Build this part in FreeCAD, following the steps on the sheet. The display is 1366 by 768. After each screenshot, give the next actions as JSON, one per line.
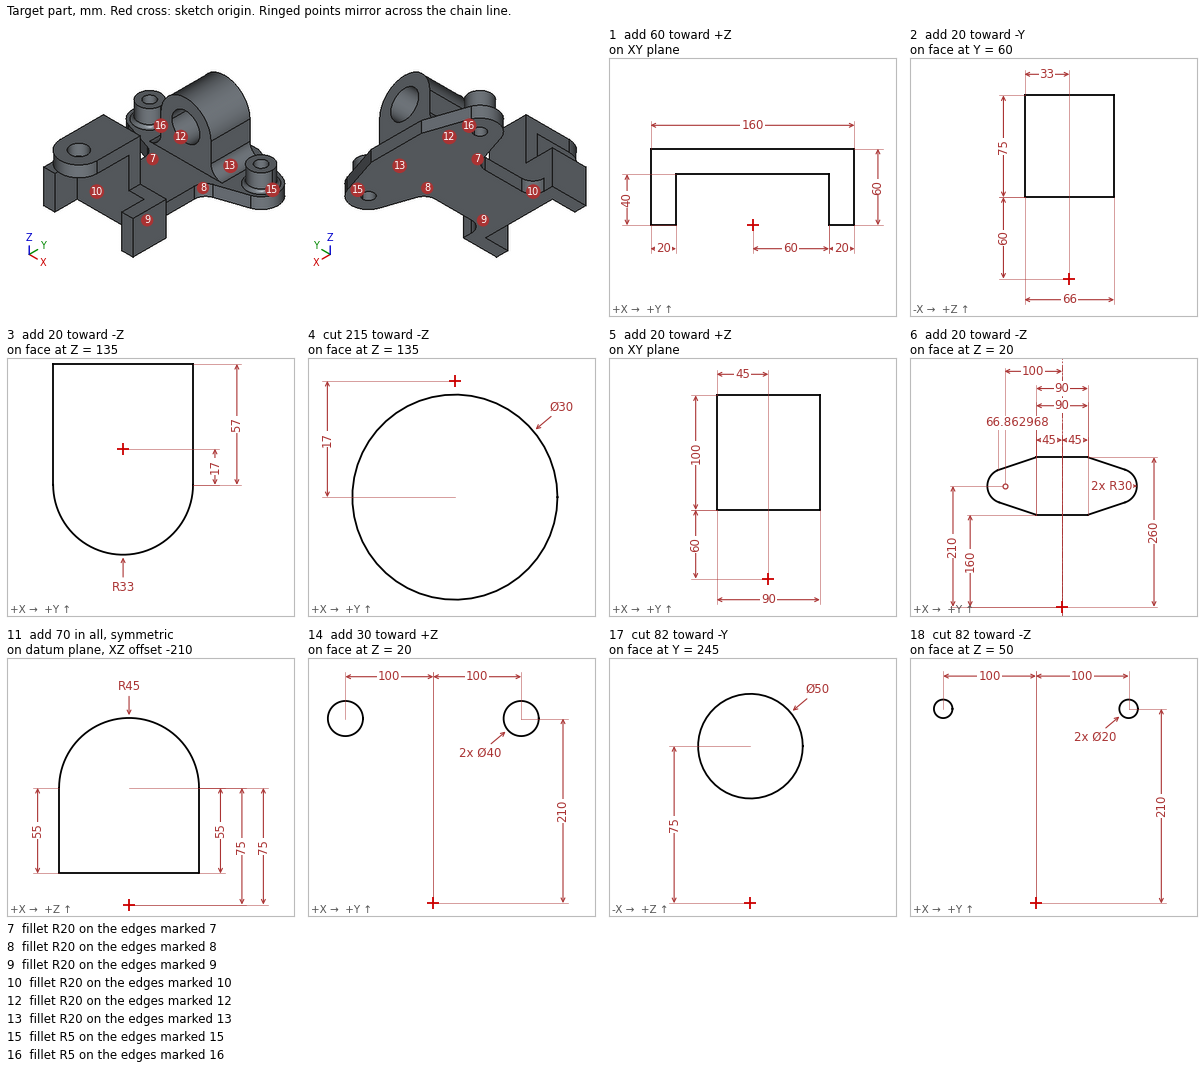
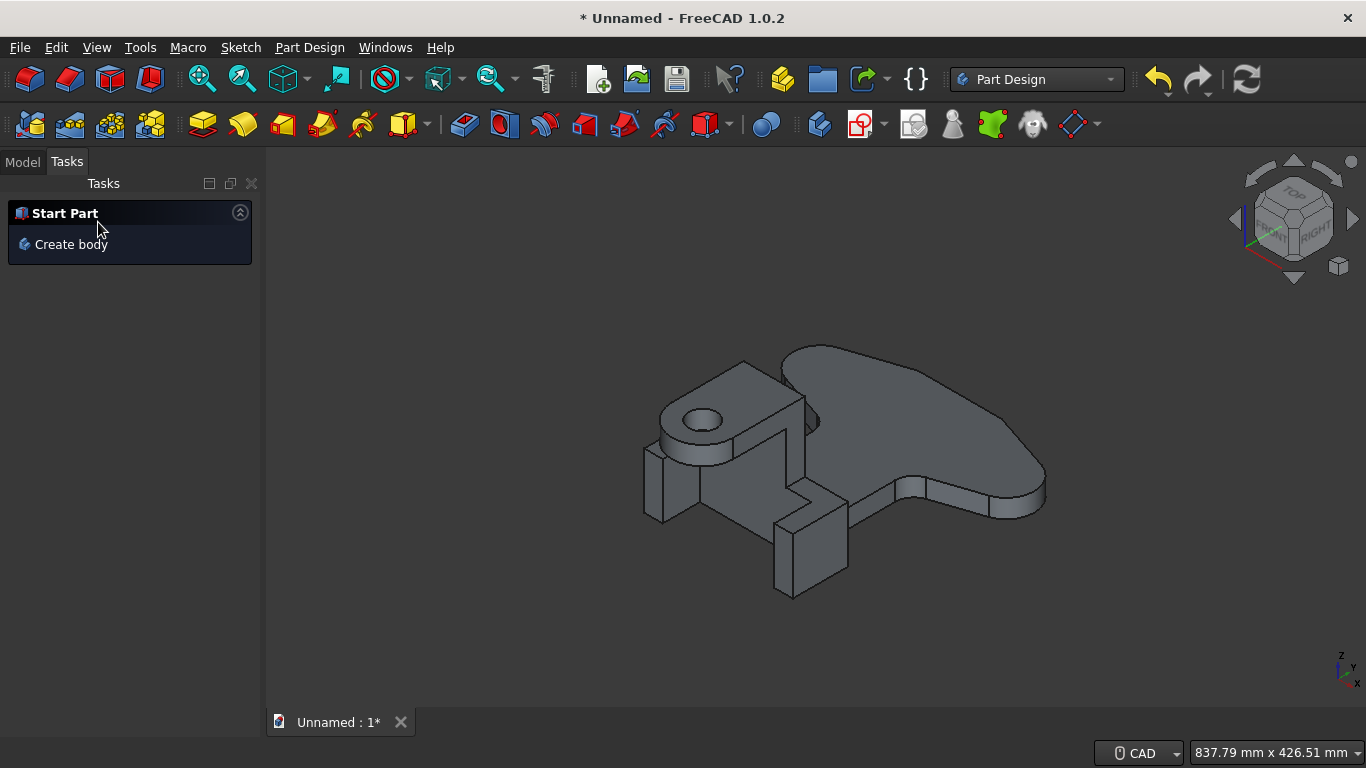
{"action": "key", "text": "2"}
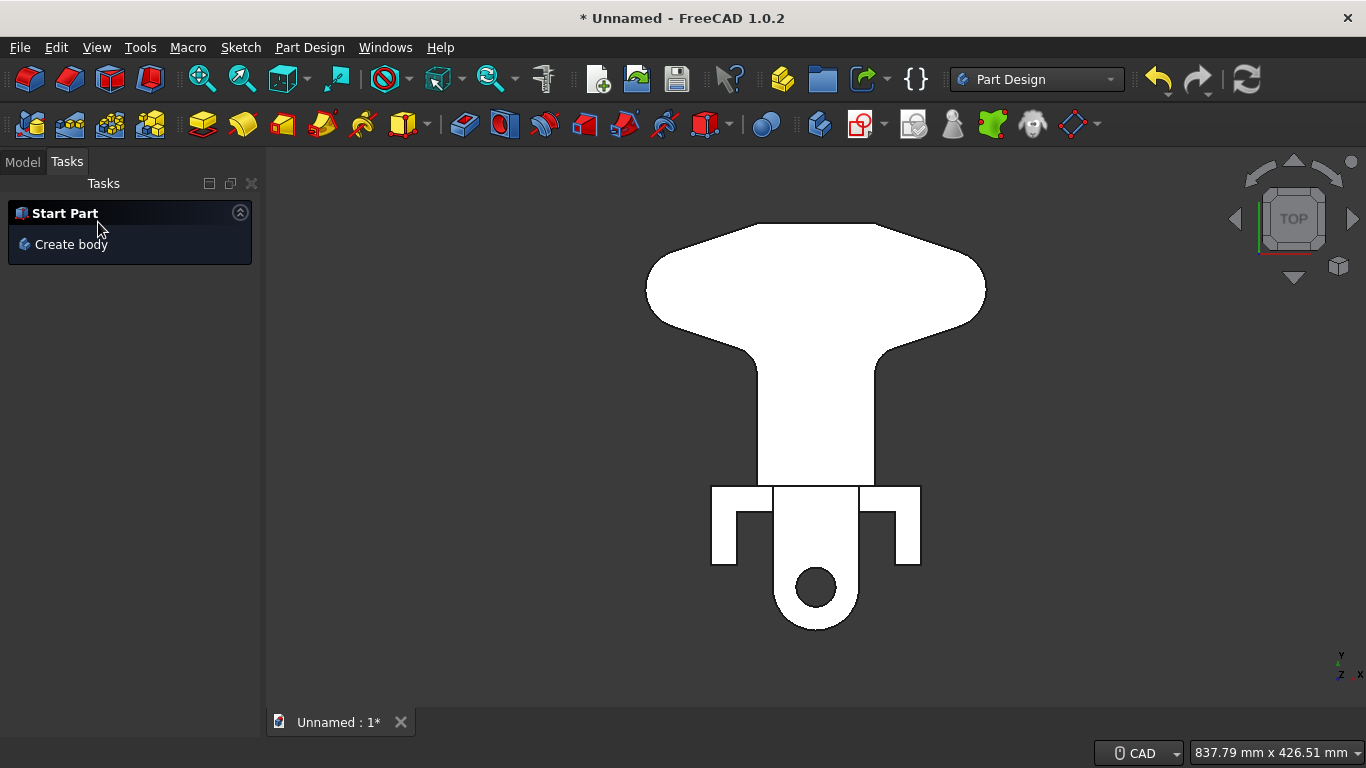
{"action": "key", "text": "0"}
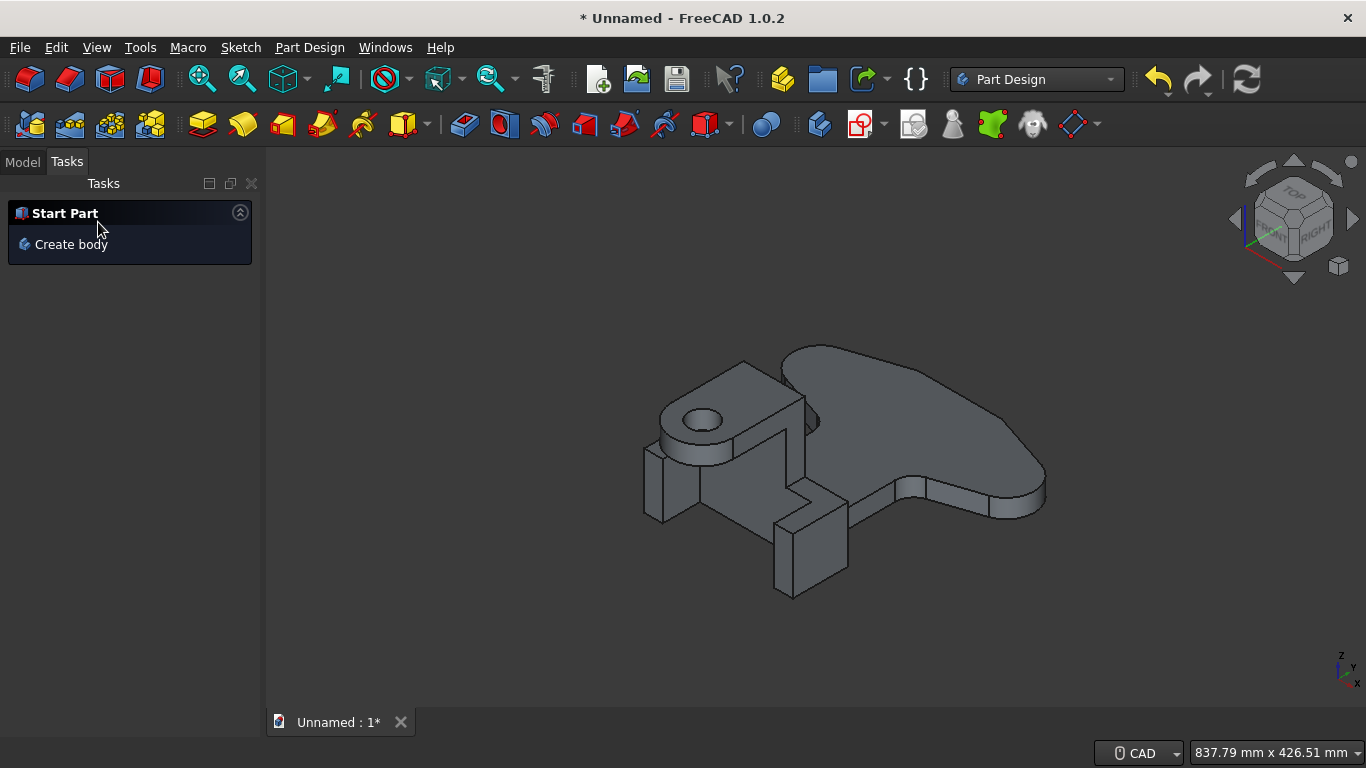
{"action": "key", "text": "1"}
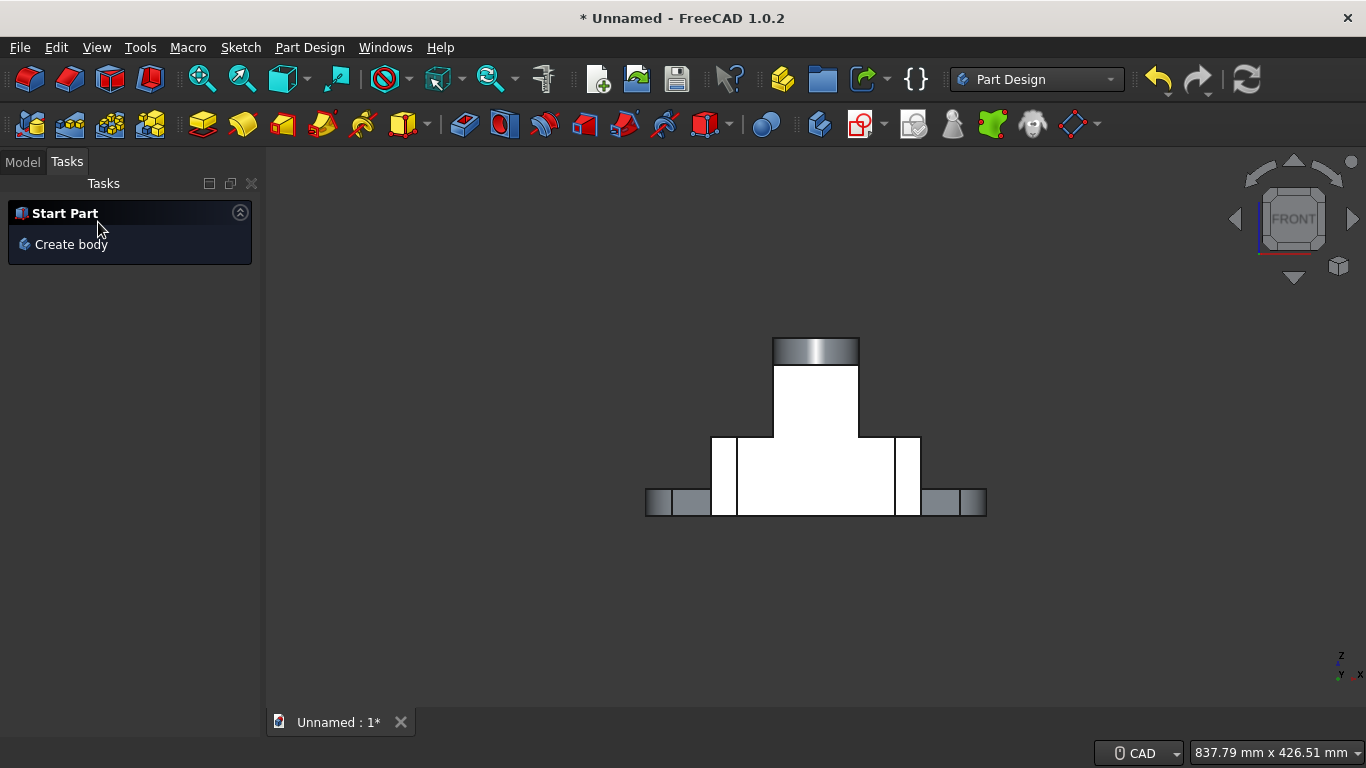
{"action": "left_click", "coordinate": [204, 80]}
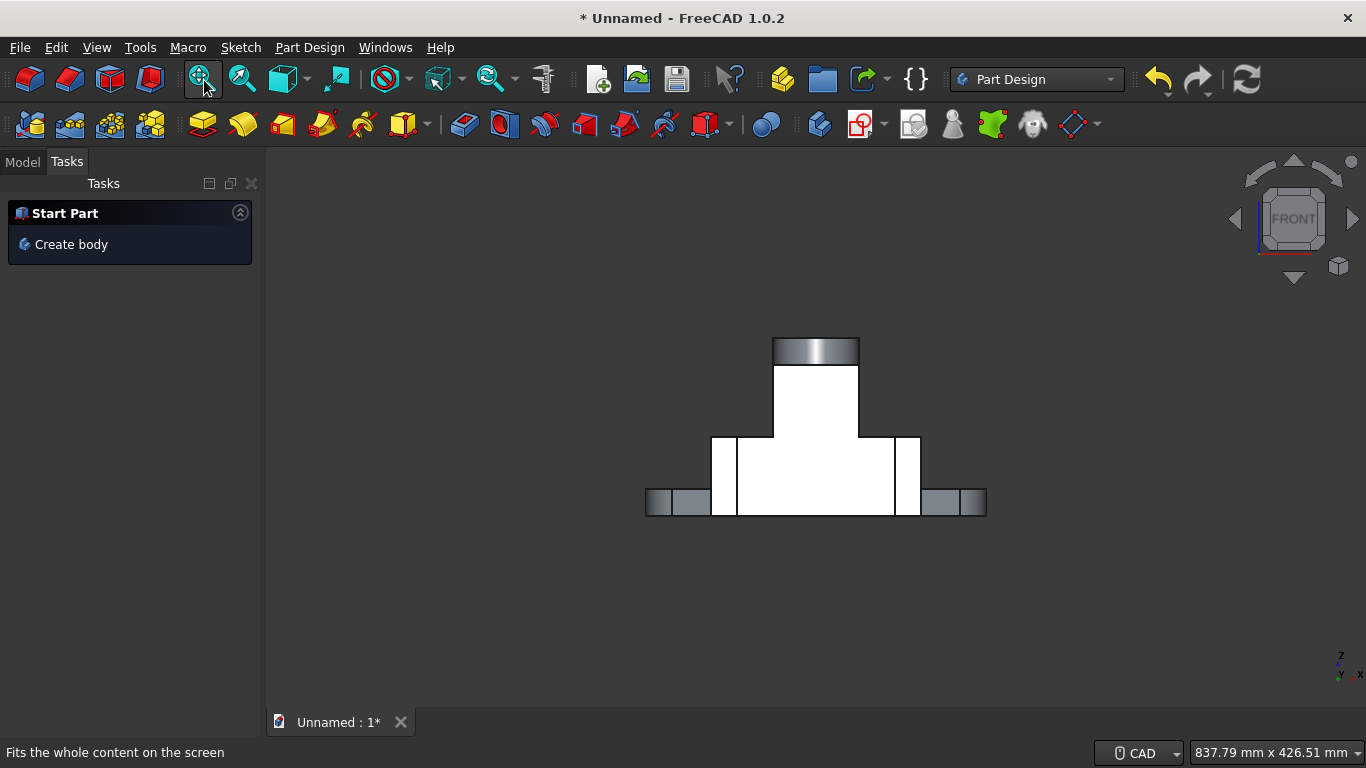
{"action": "key", "text": "3"}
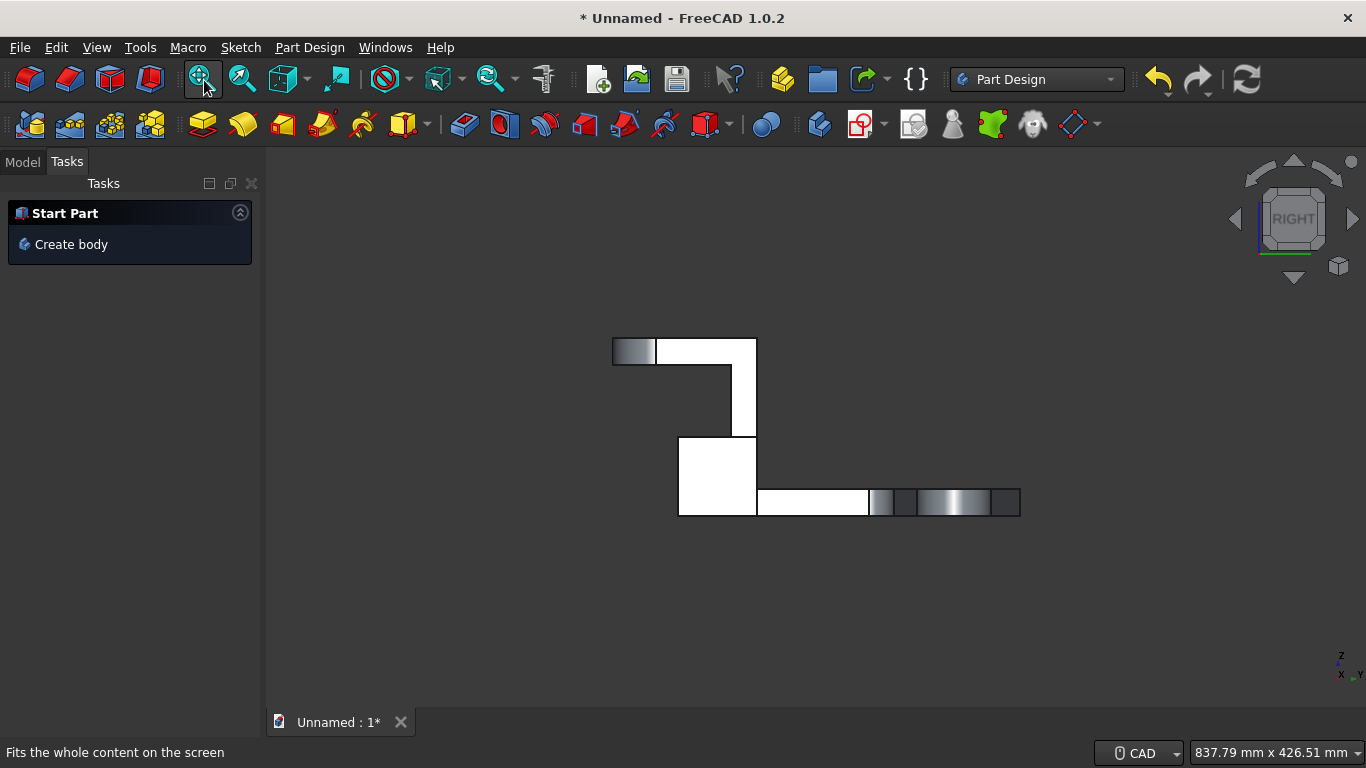
{"action": "key", "text": "v f"}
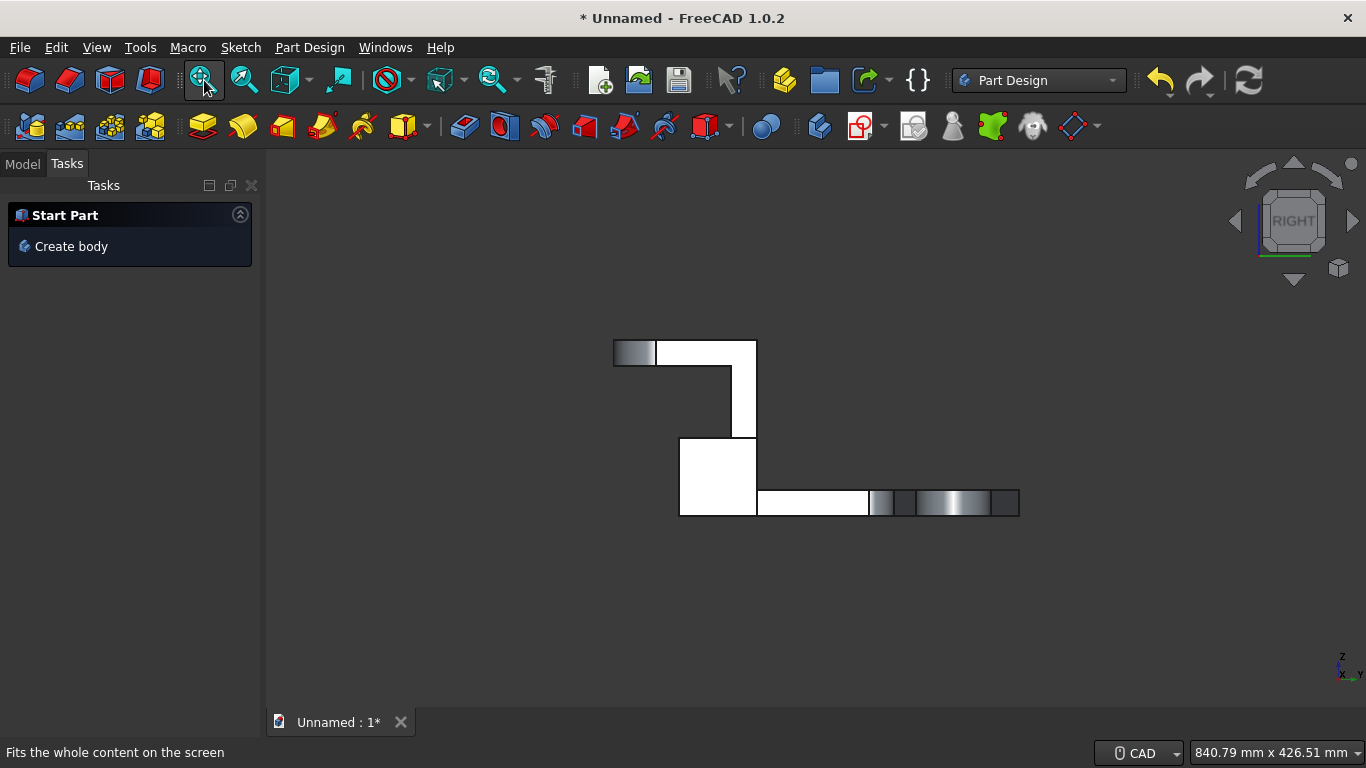
{"action": "key", "text": "5"}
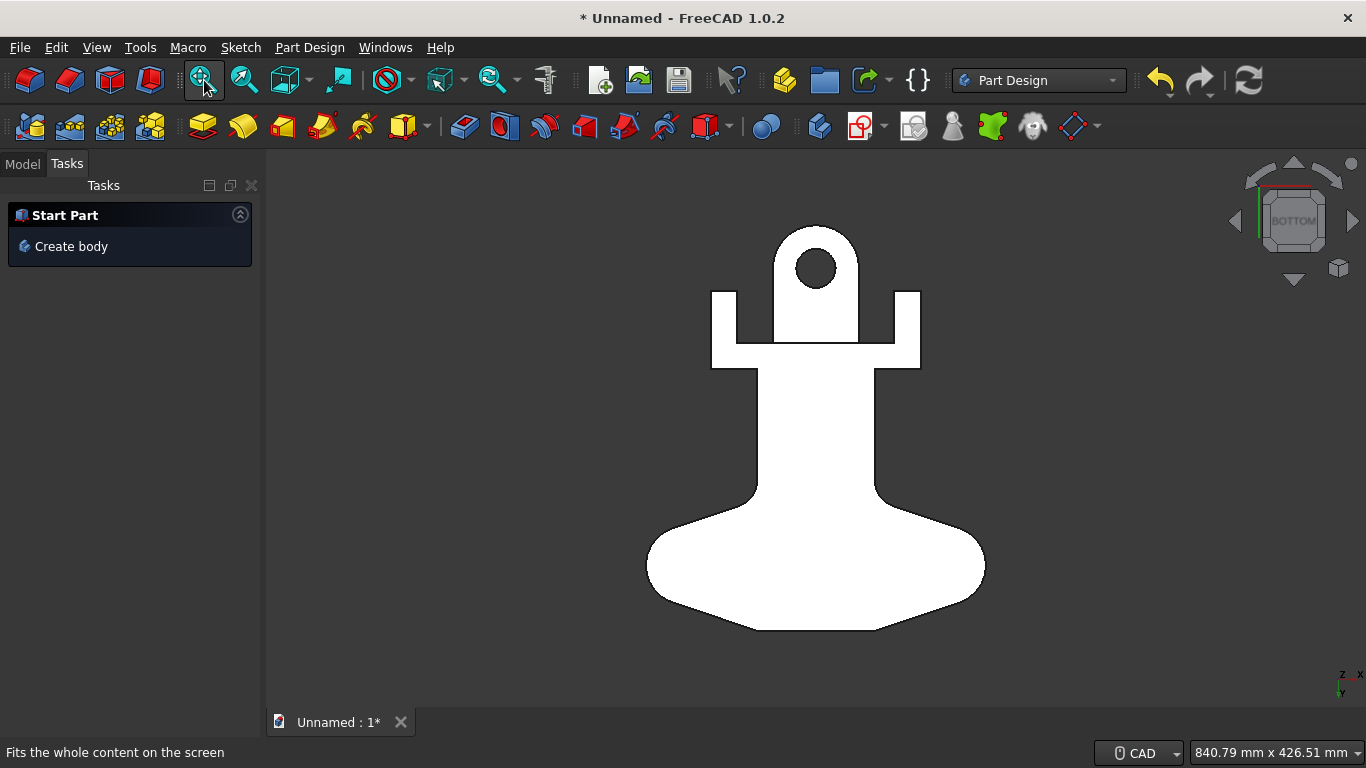
{"action": "key", "text": "4"}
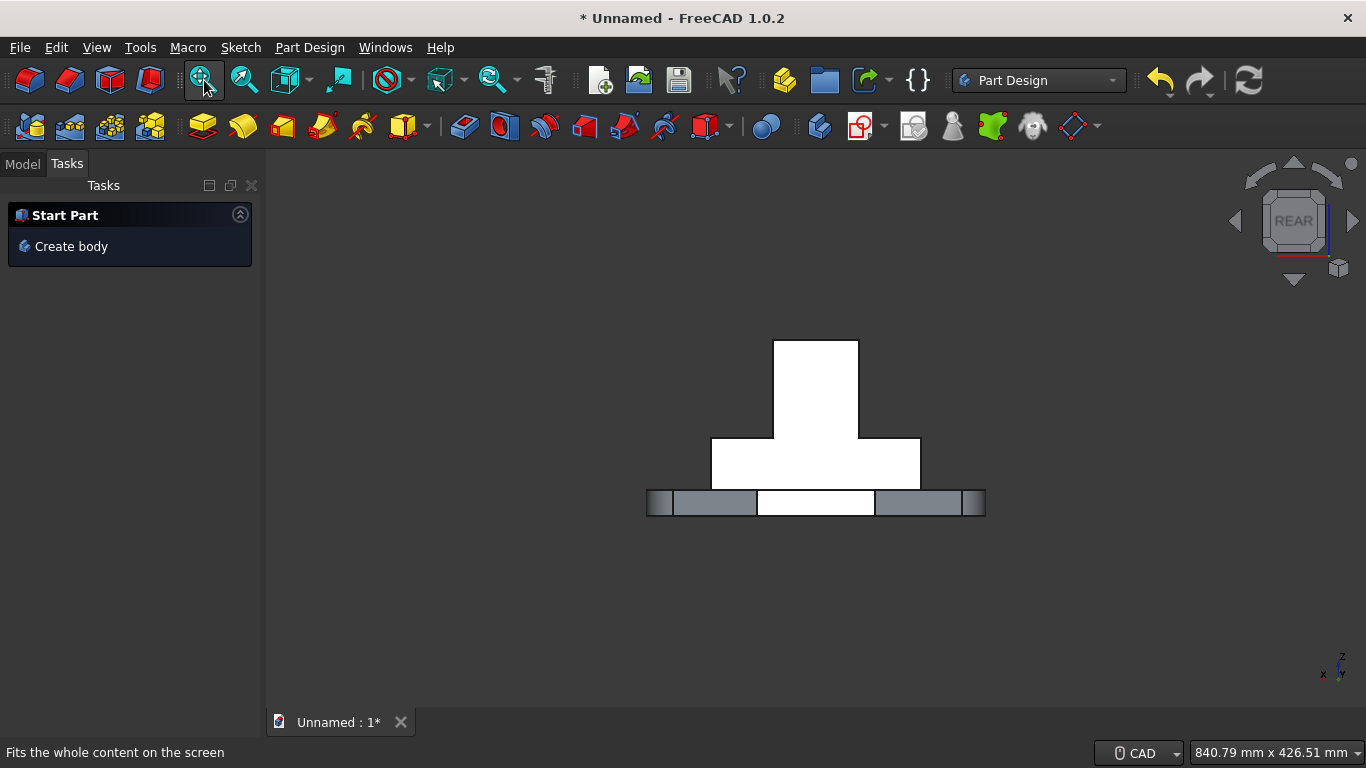
{"action": "key", "text": "v f"}